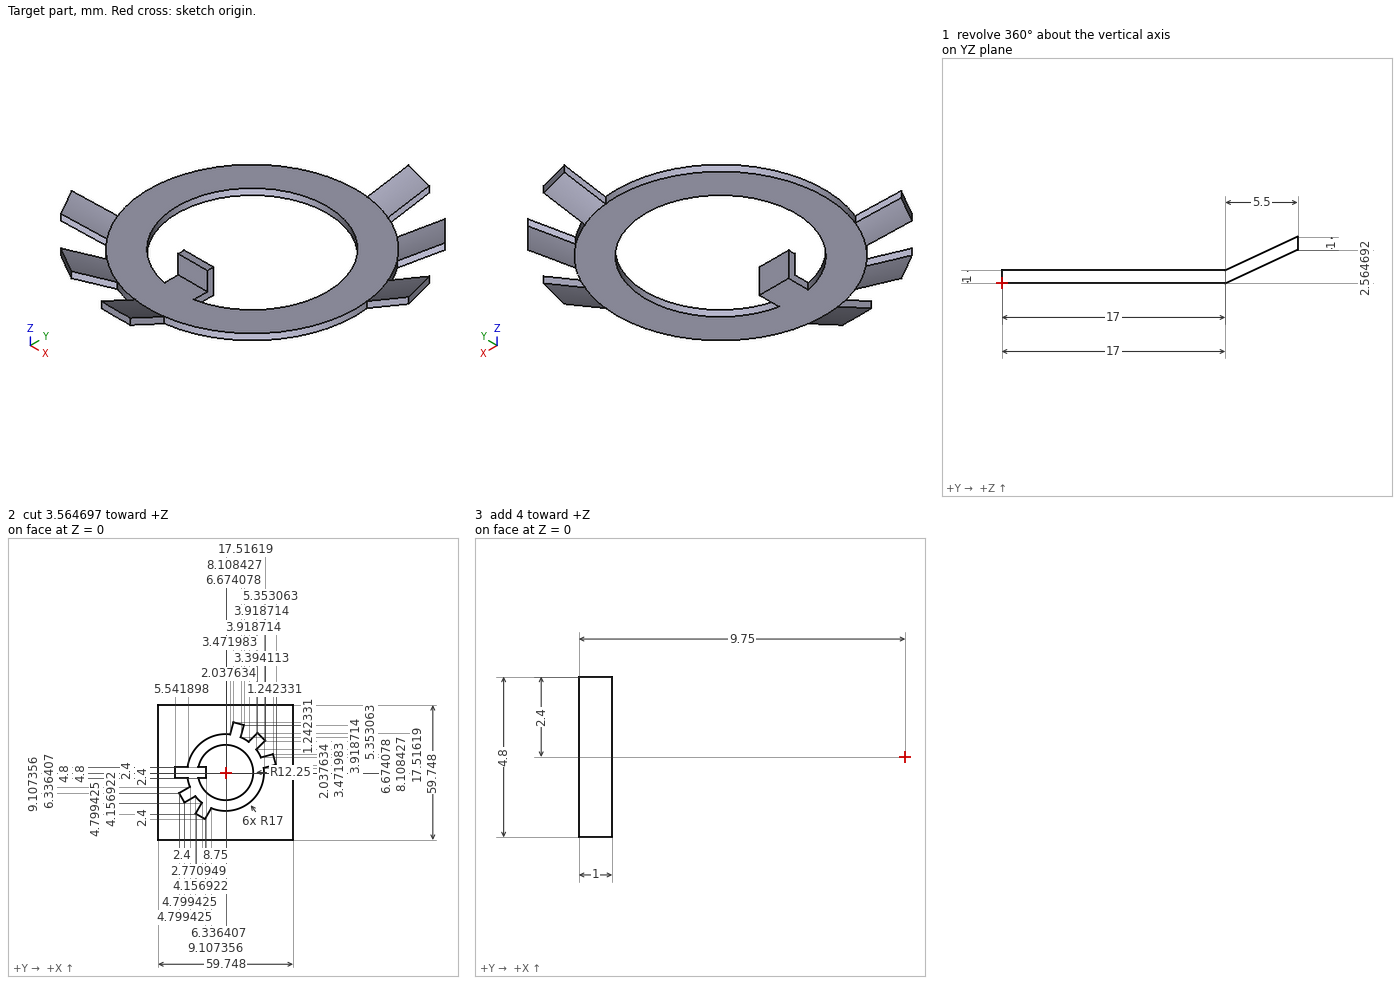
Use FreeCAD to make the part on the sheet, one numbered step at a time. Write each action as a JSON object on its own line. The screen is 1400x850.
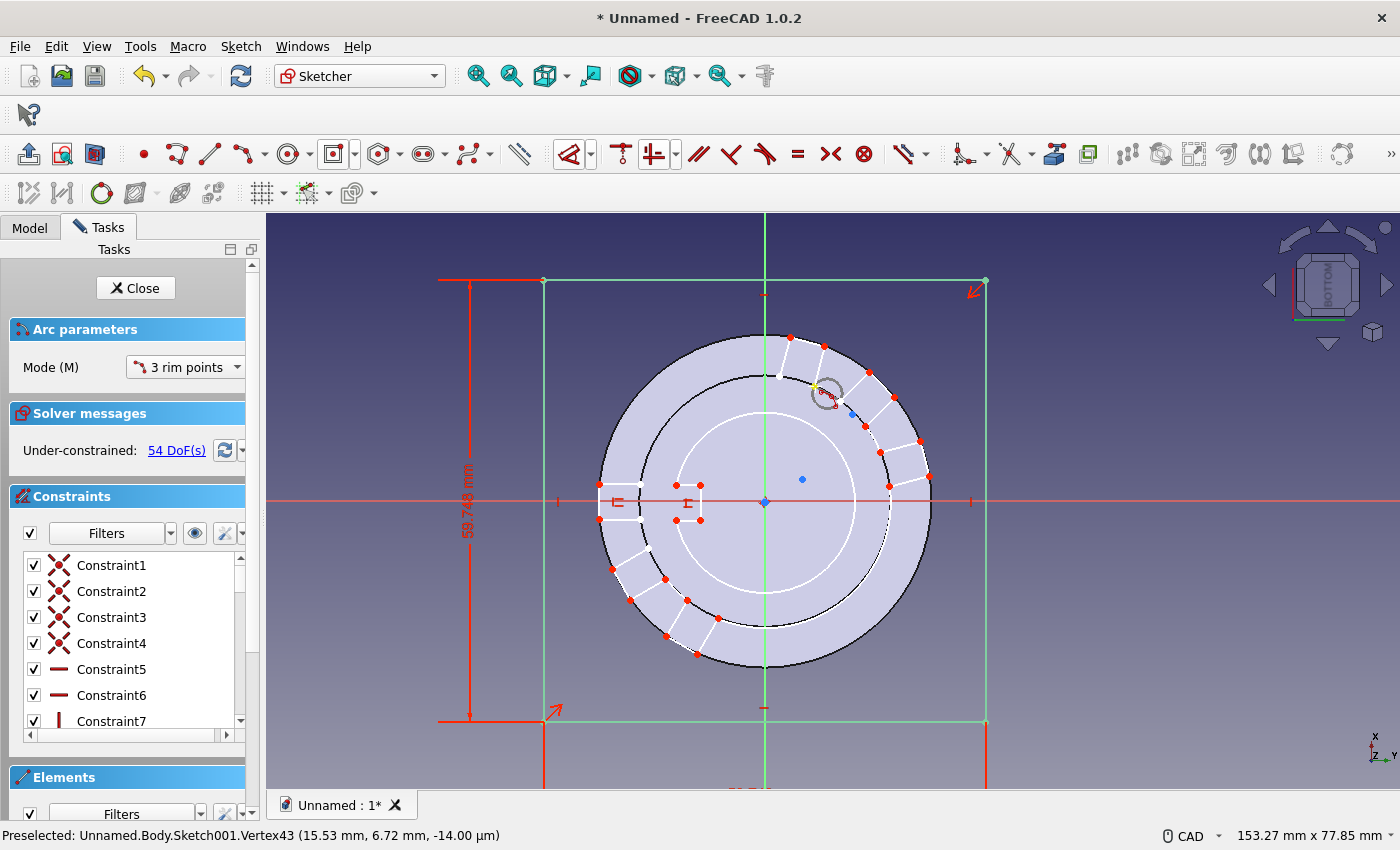
{"action": "scroll", "coordinate": [828, 392], "scroll_direction": "up", "scroll_amount": 15}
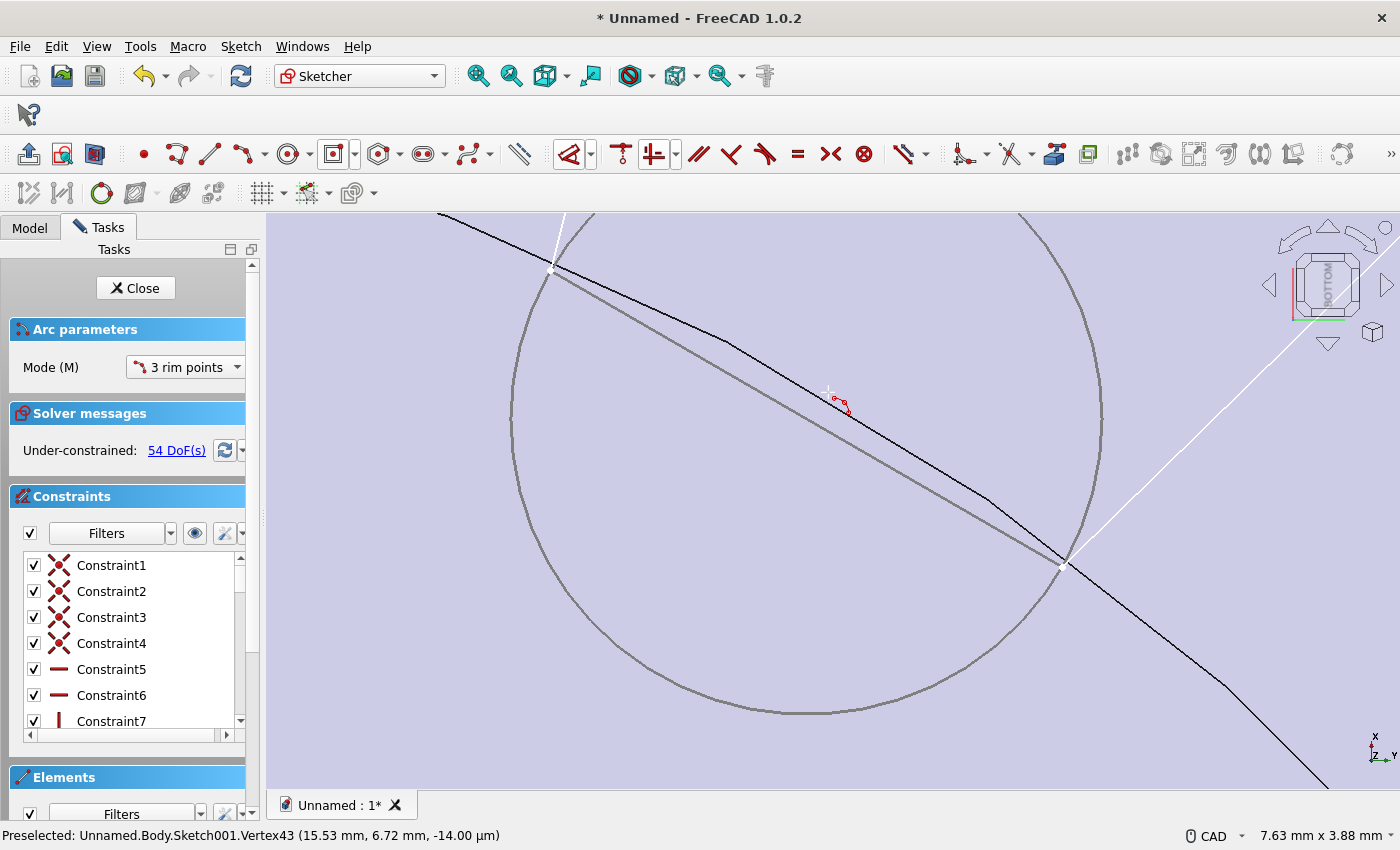
{"action": "left_click", "coordinate": [815, 391]}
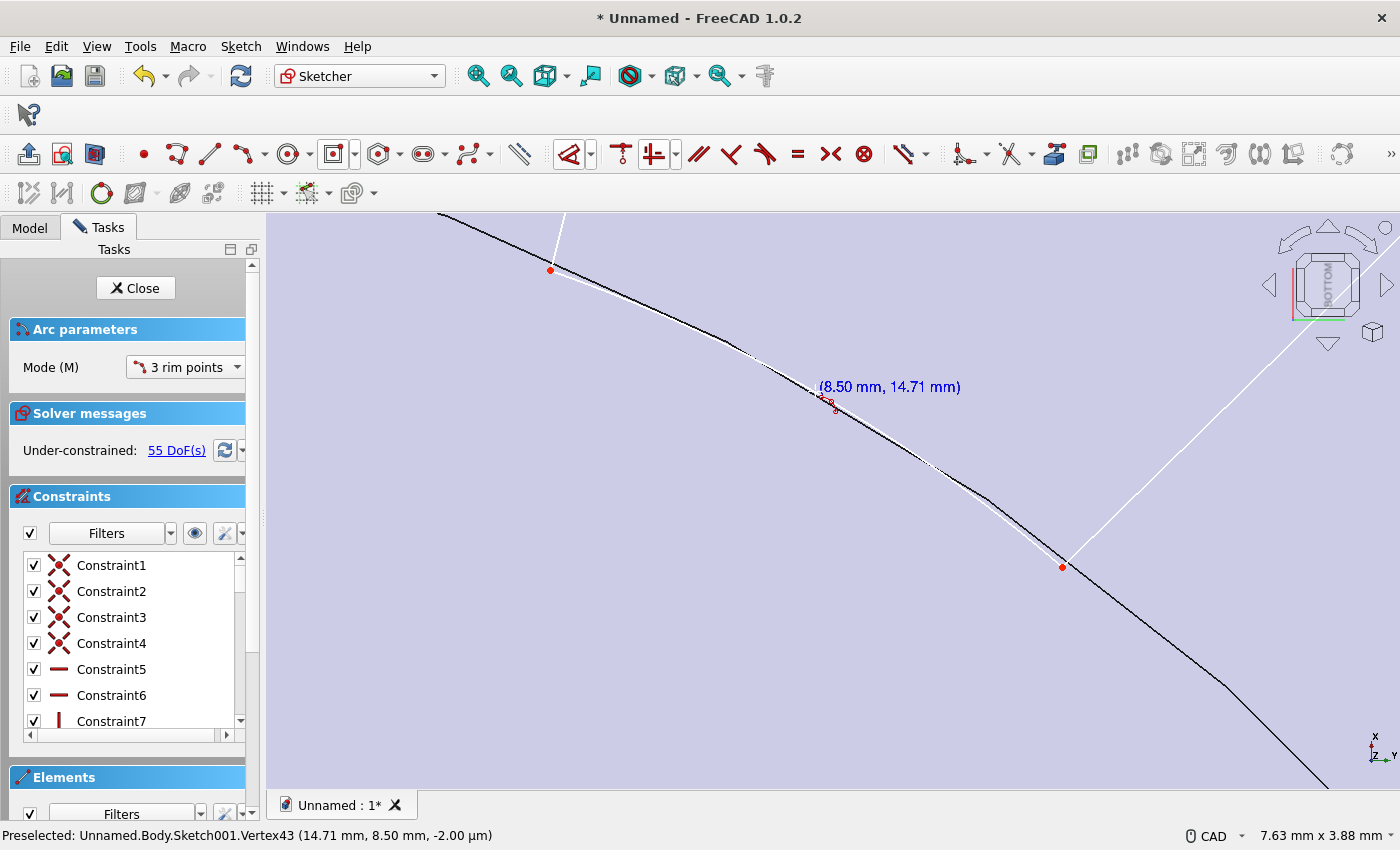
{"action": "scroll", "coordinate": [828, 392], "scroll_direction": "down", "scroll_amount": 15}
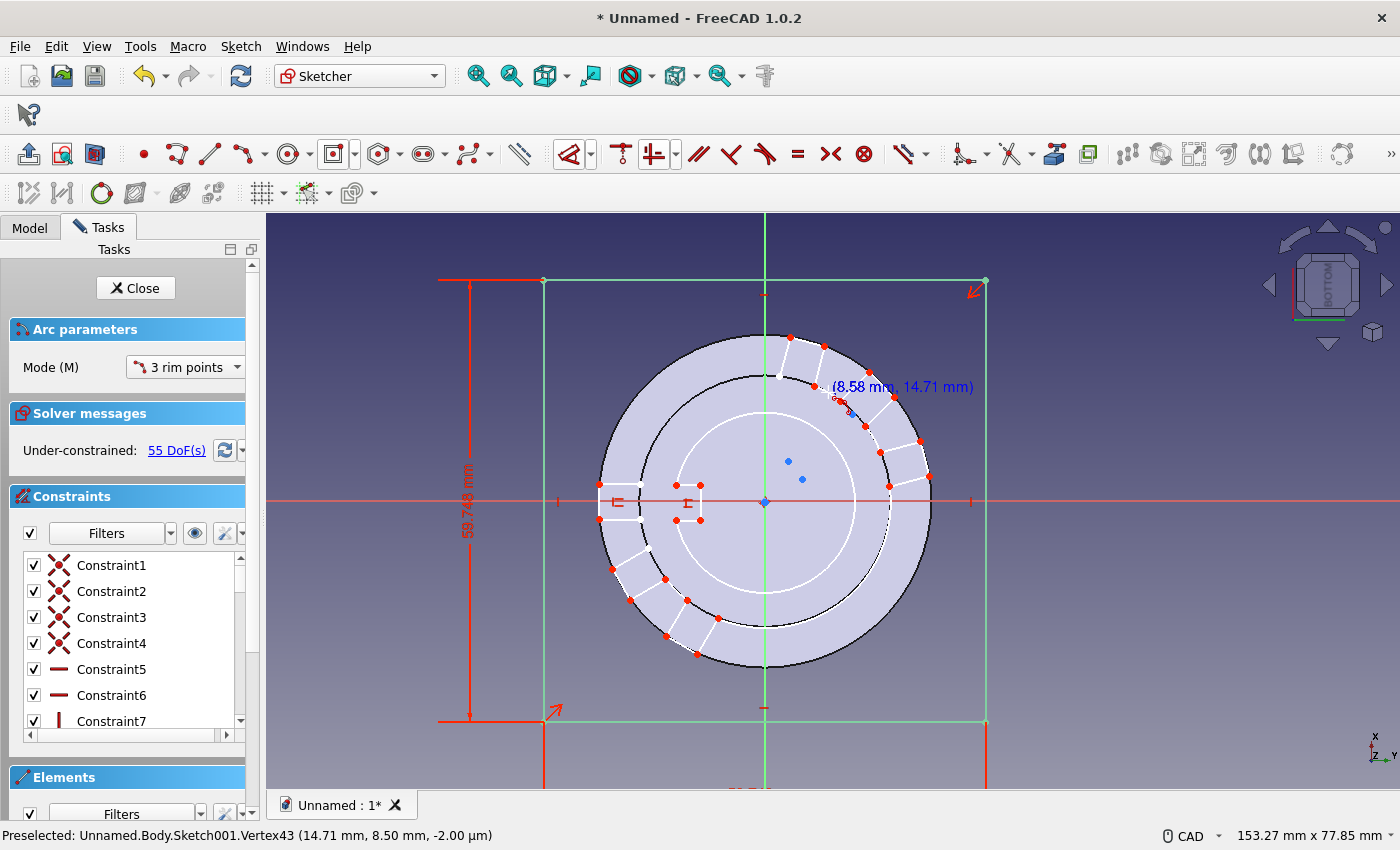
{"action": "left_click", "coordinate": [780, 377]}
{"action": "left_click", "coordinate": [640, 484]}
{"action": "left_click", "coordinate": [688, 401]}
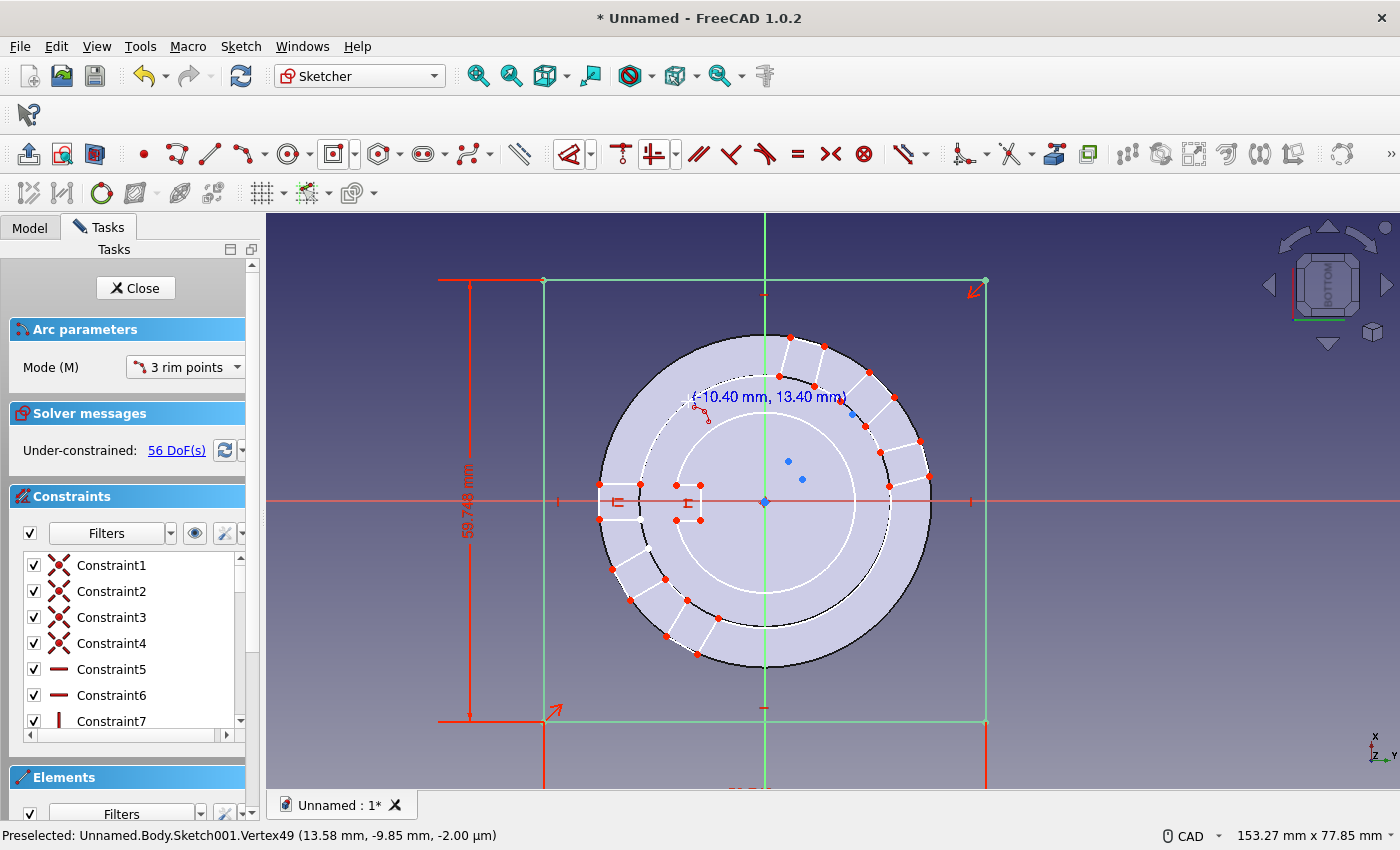
{"action": "left_click", "coordinate": [640, 520]}
{"action": "left_click", "coordinate": [648, 548]}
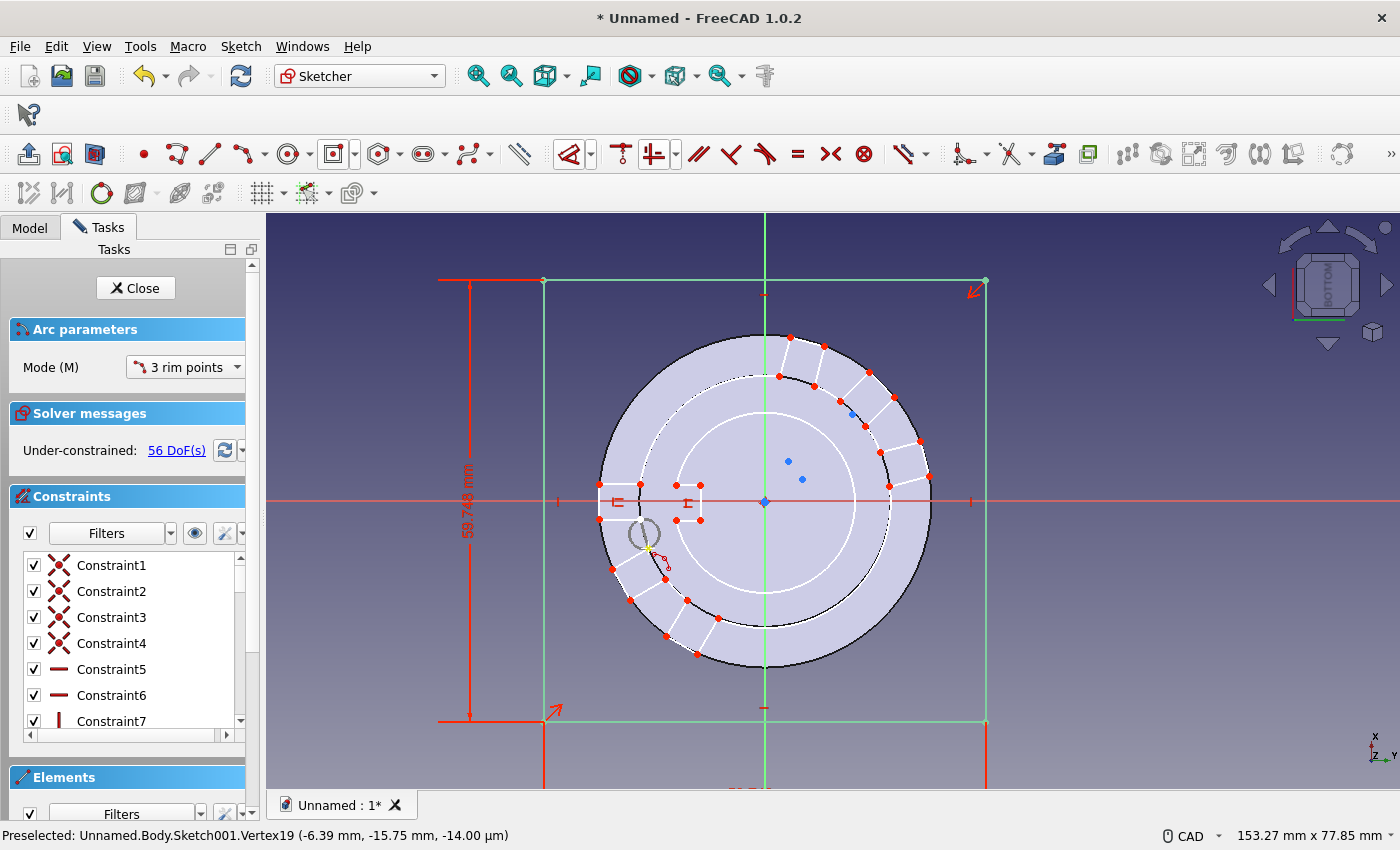
{"action": "scroll", "coordinate": [643, 534], "scroll_direction": "up", "scroll_amount": 15}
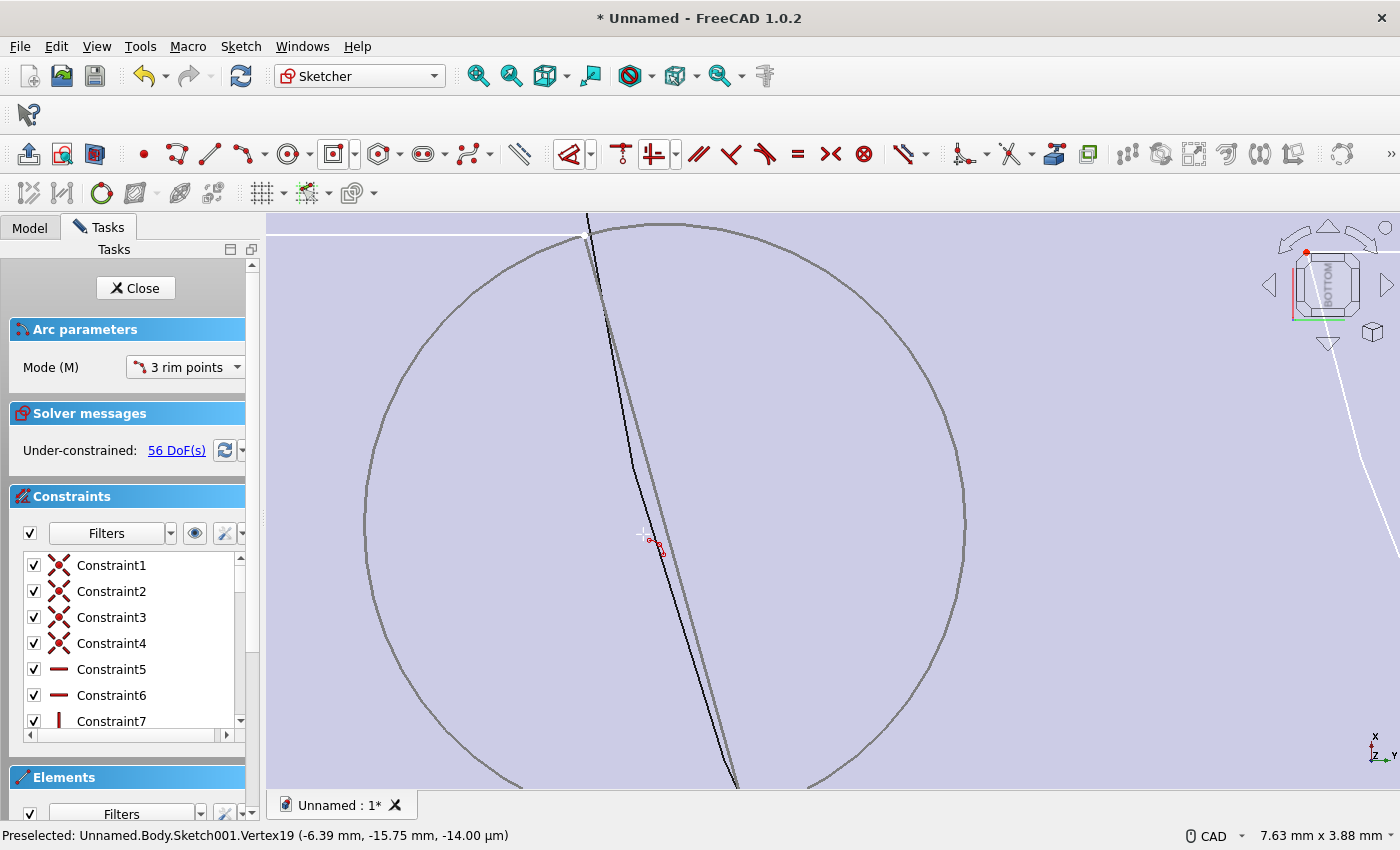
{"action": "left_click", "coordinate": [646, 518]}
{"action": "key", "text": "Escape"}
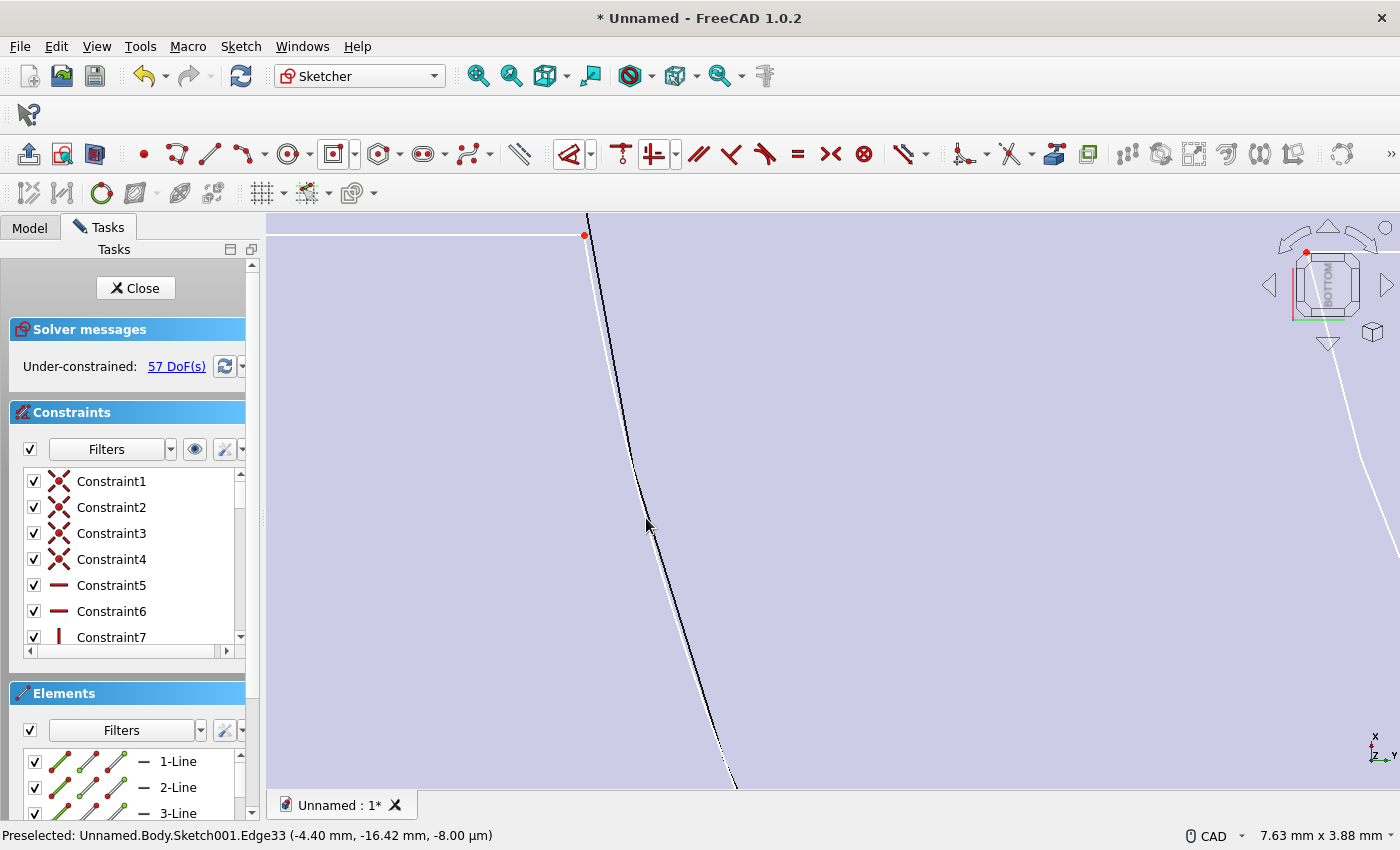
{"action": "scroll", "coordinate": [643, 534], "scroll_direction": "down", "scroll_amount": 15}